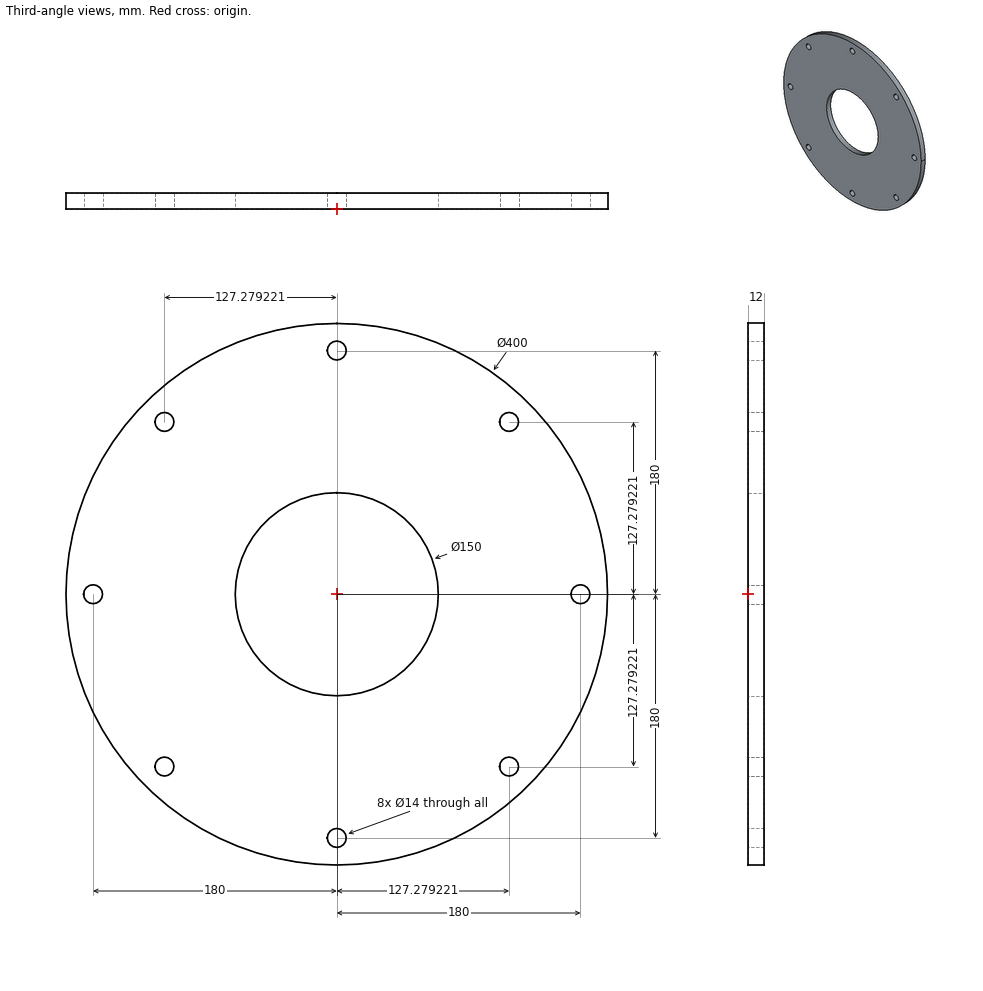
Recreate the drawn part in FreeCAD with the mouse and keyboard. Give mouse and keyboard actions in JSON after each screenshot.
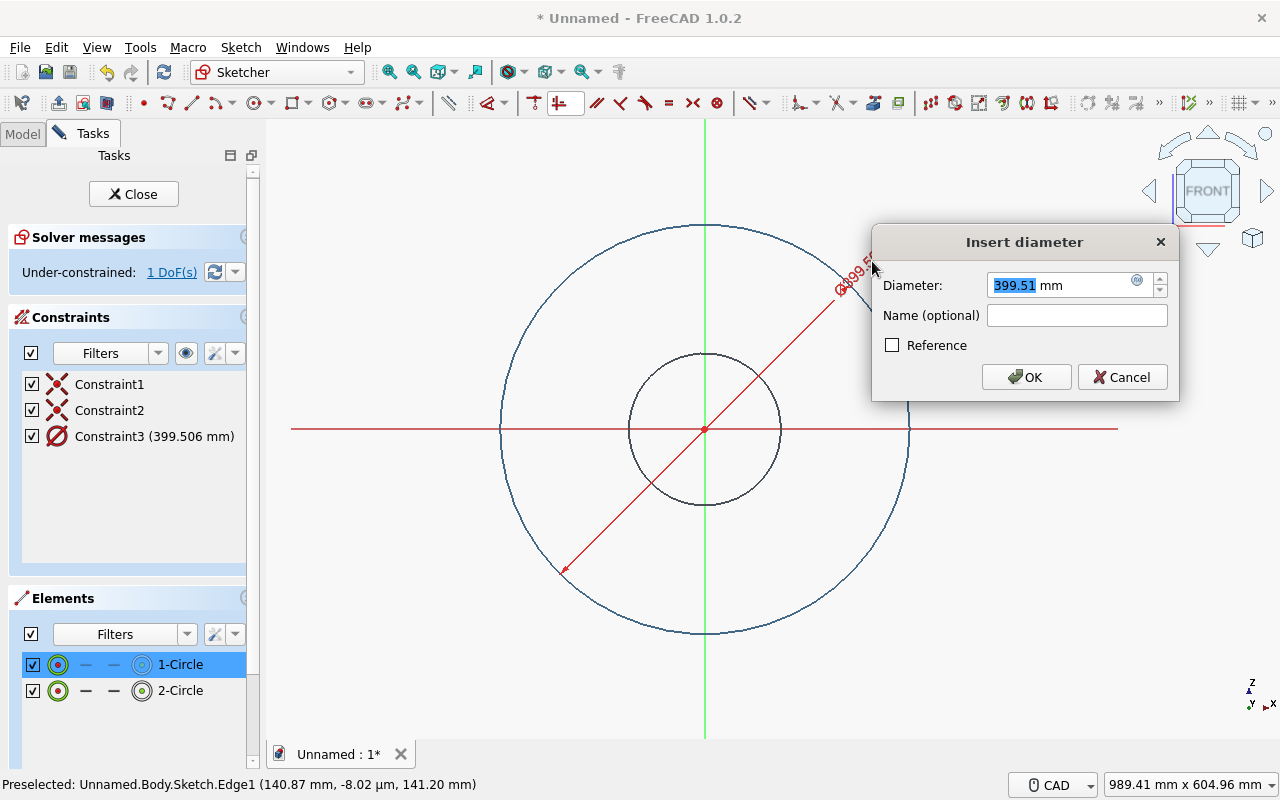
{"action": "type", "text": "400"}
{"action": "key", "text": "Return"}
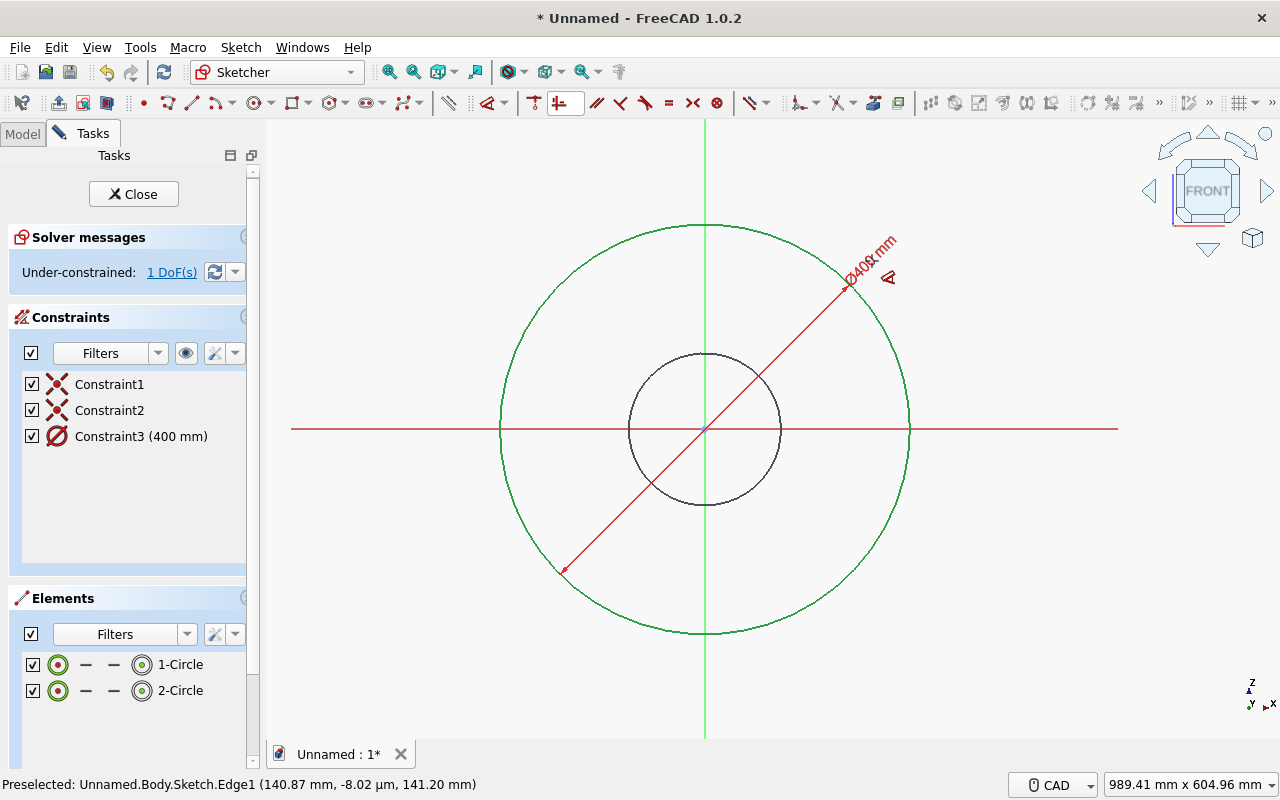
{"action": "left_click", "coordinate": [758, 375]}
{"action": "left_click", "coordinate": [780, 352]}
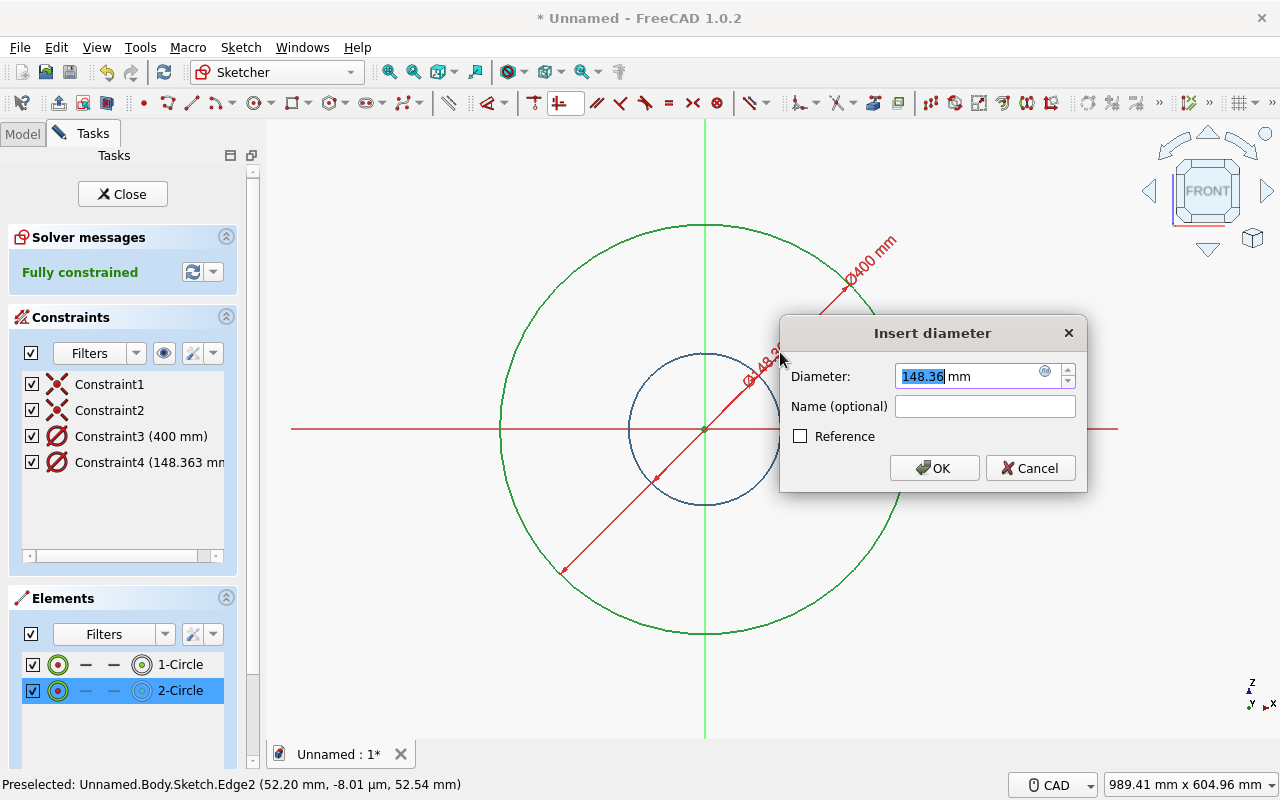
{"action": "type", "text": "150"}
{"action": "key", "text": "Return"}
{"action": "key", "text": "Escape"}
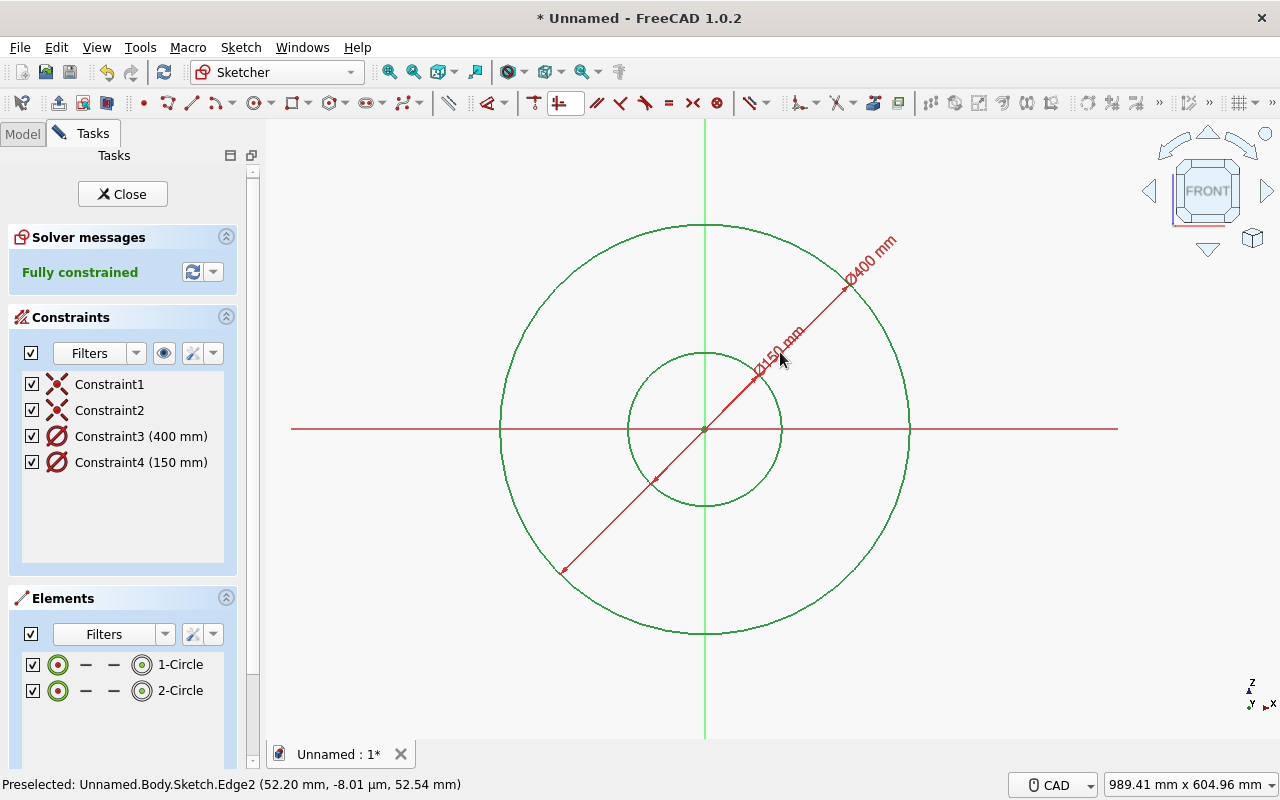
{"action": "left_click", "coordinate": [123, 194]}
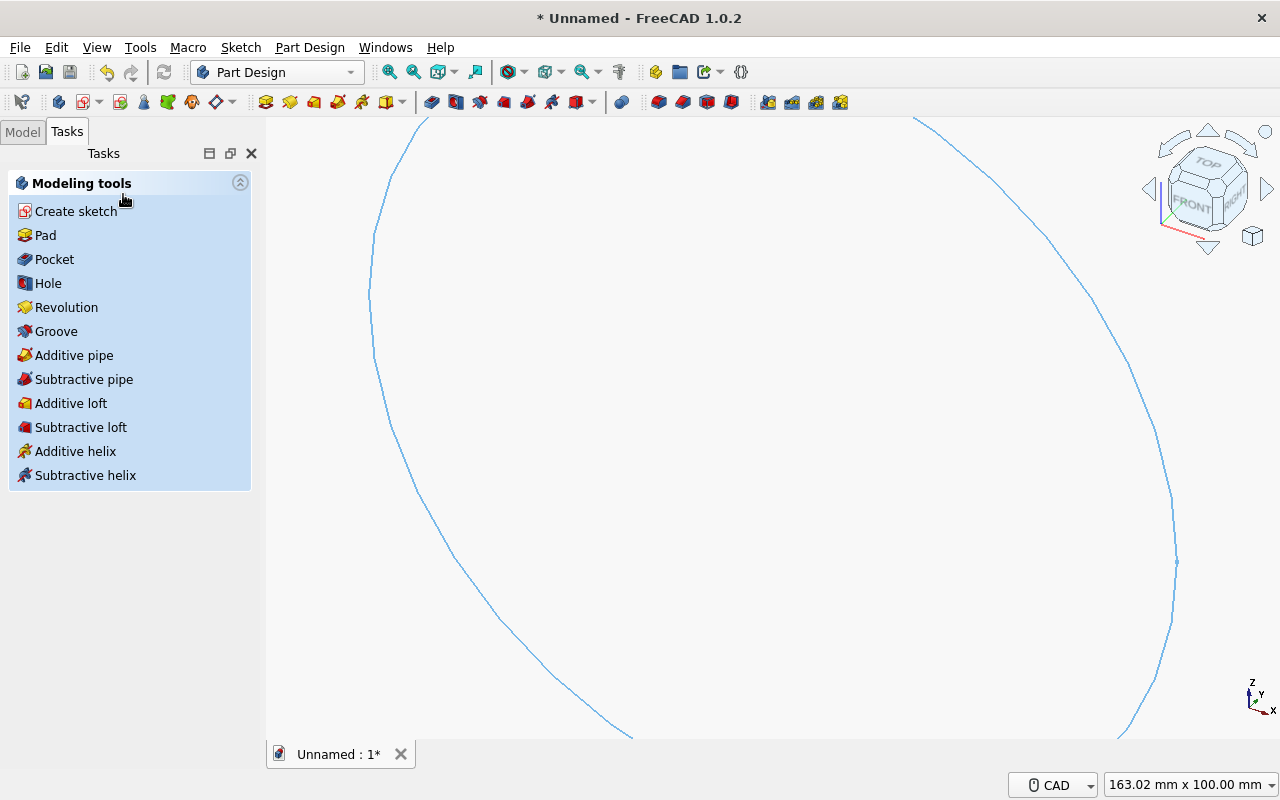
{"action": "left_click", "coordinate": [266, 102]}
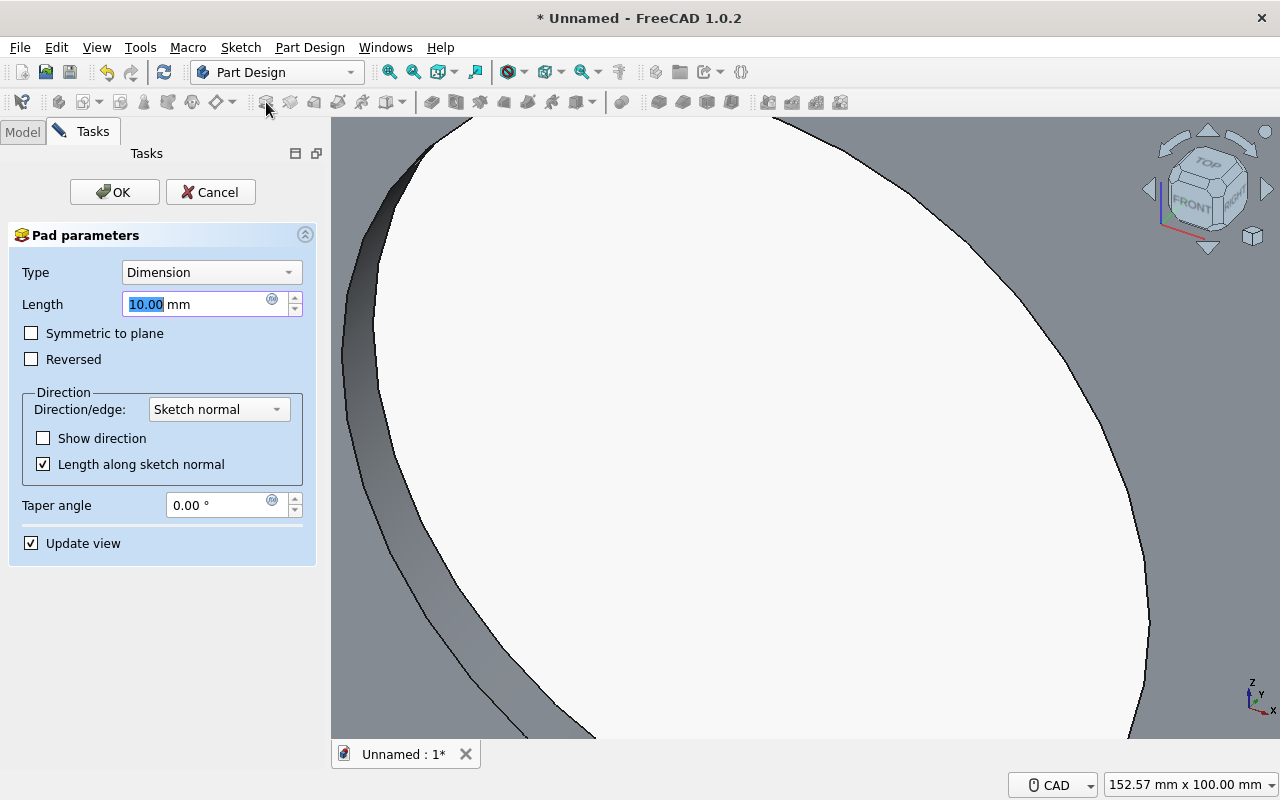
{"action": "type", "text": "12"}
{"action": "key", "text": "Tab"}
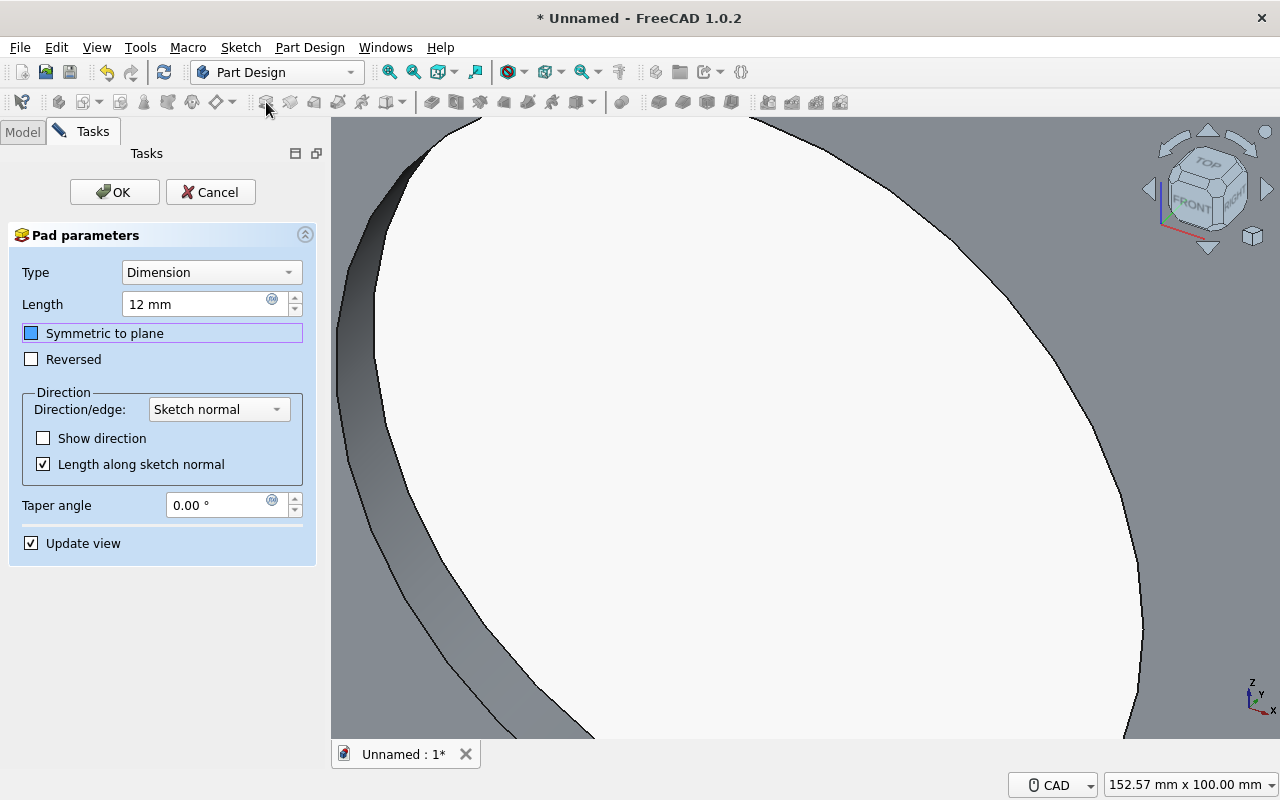
{"action": "left_click", "coordinate": [30, 359]}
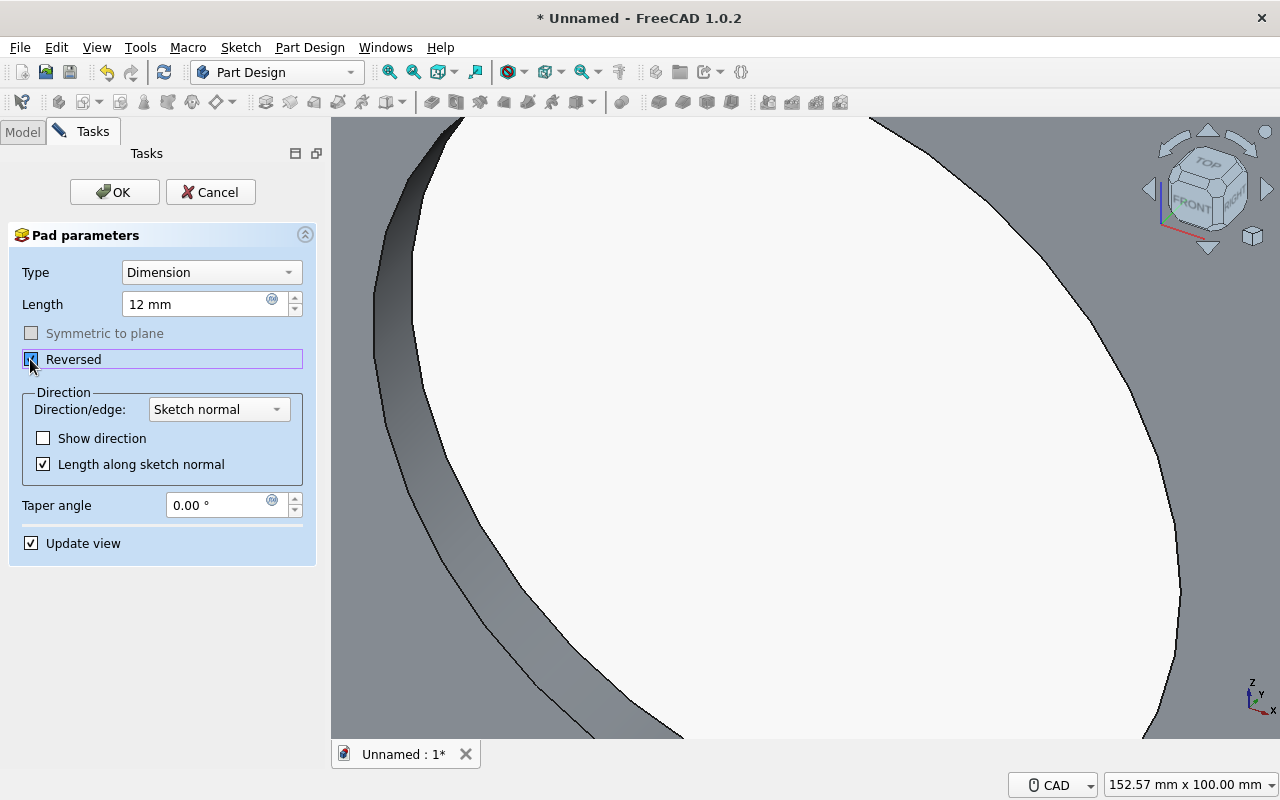
{"action": "left_click", "coordinate": [115, 192]}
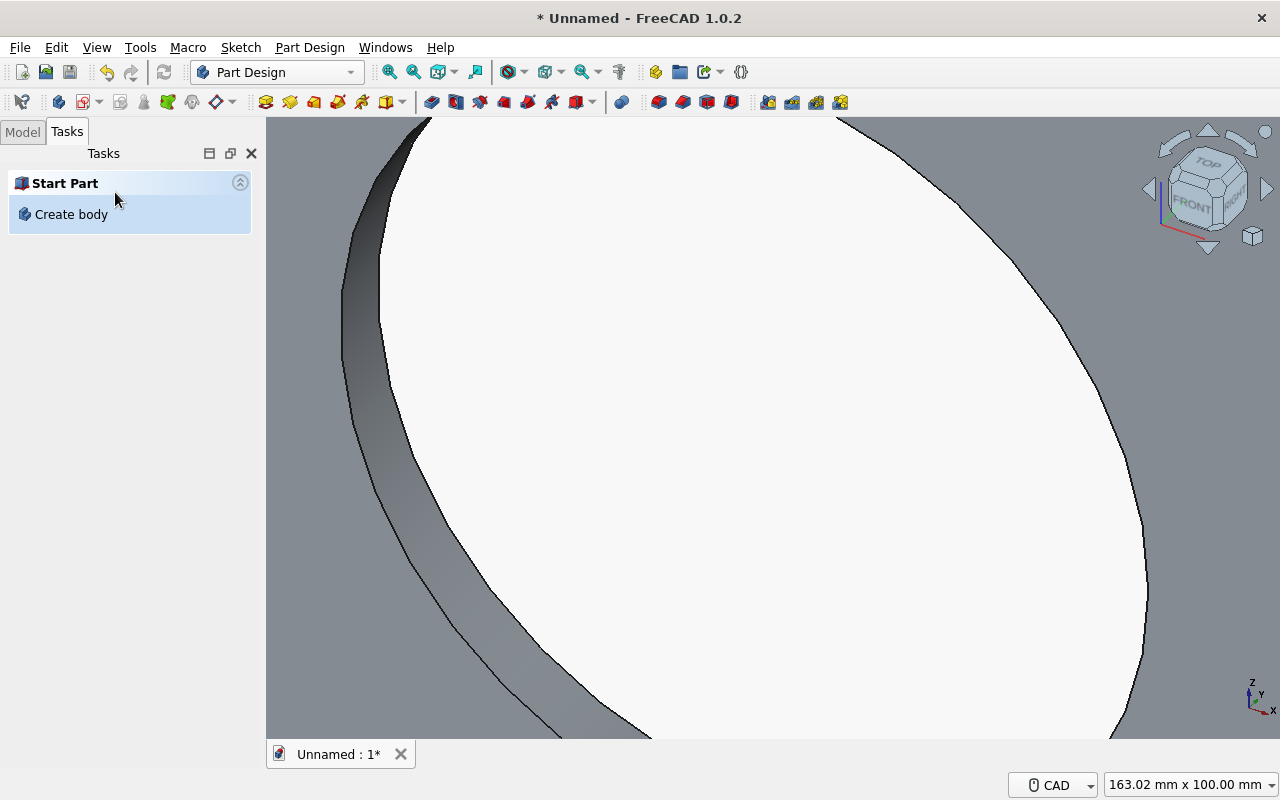
{"action": "left_click", "coordinate": [390, 72]}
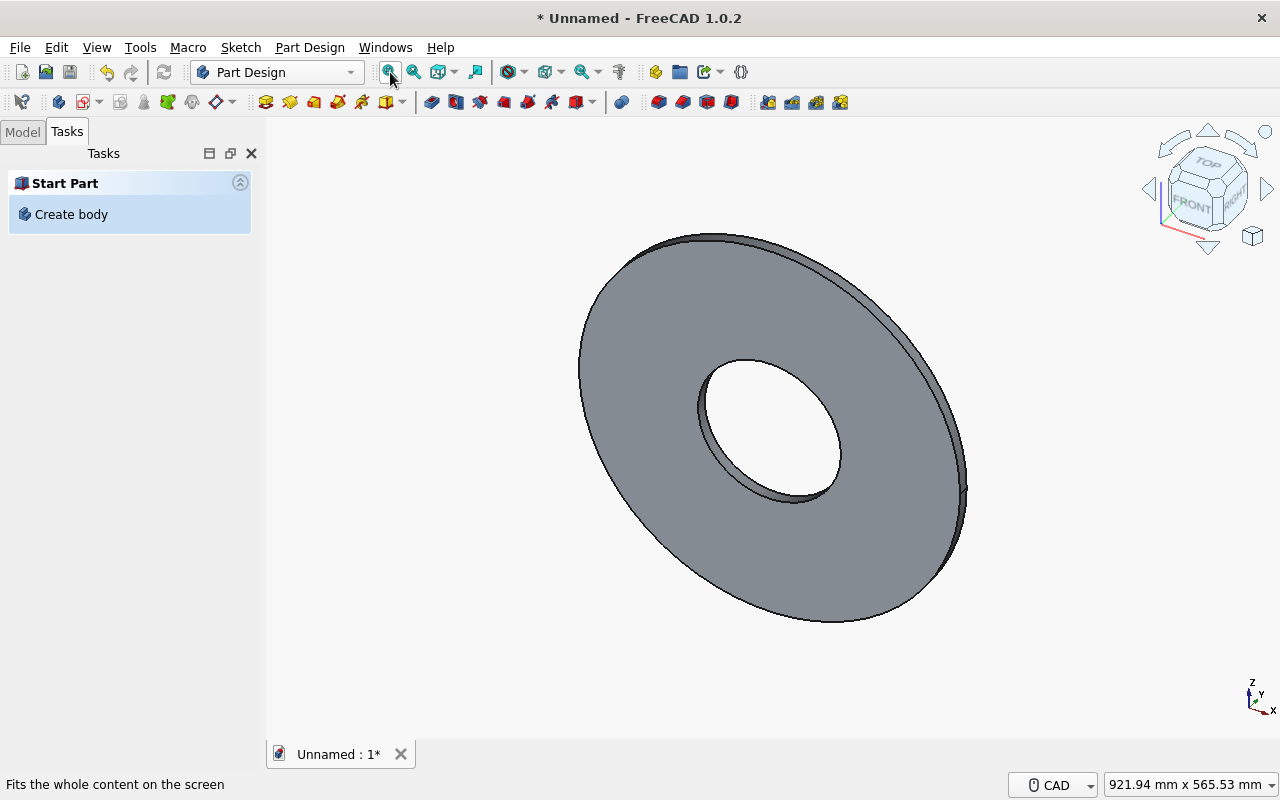
{"action": "key", "text": "4"}